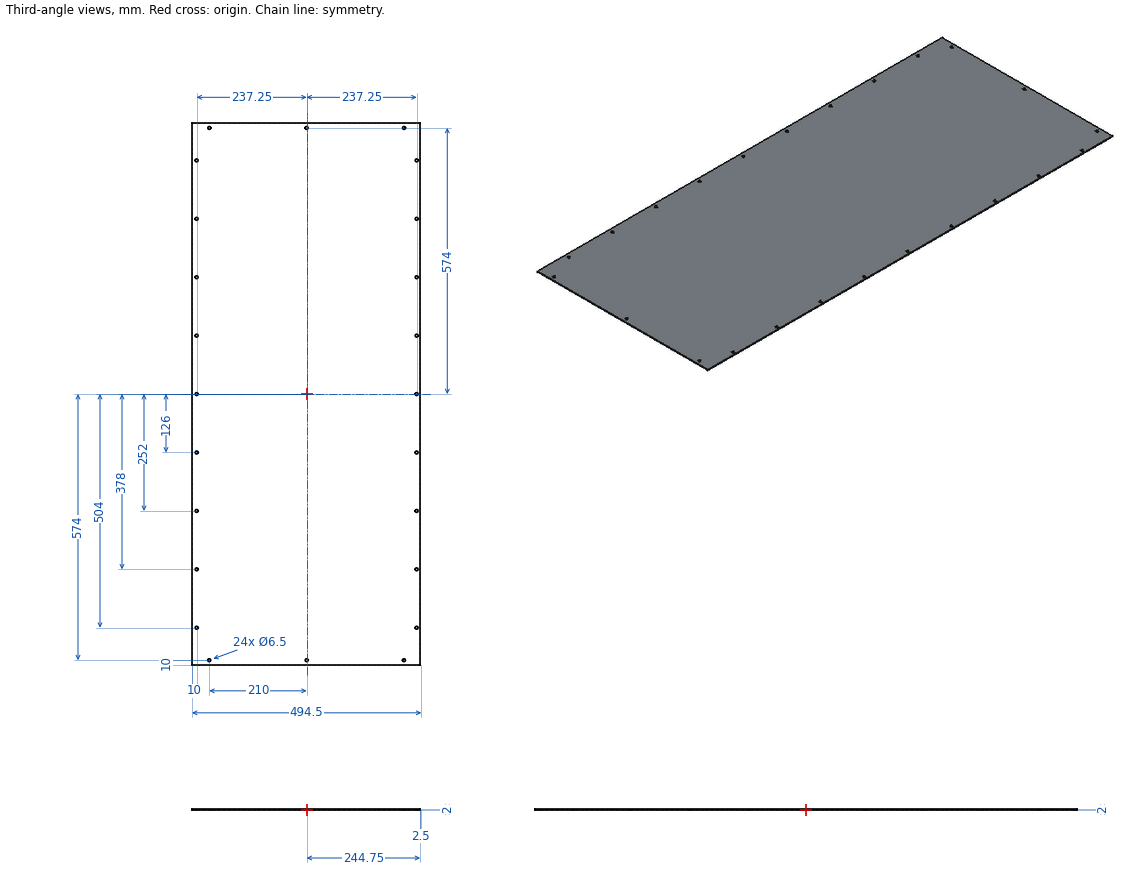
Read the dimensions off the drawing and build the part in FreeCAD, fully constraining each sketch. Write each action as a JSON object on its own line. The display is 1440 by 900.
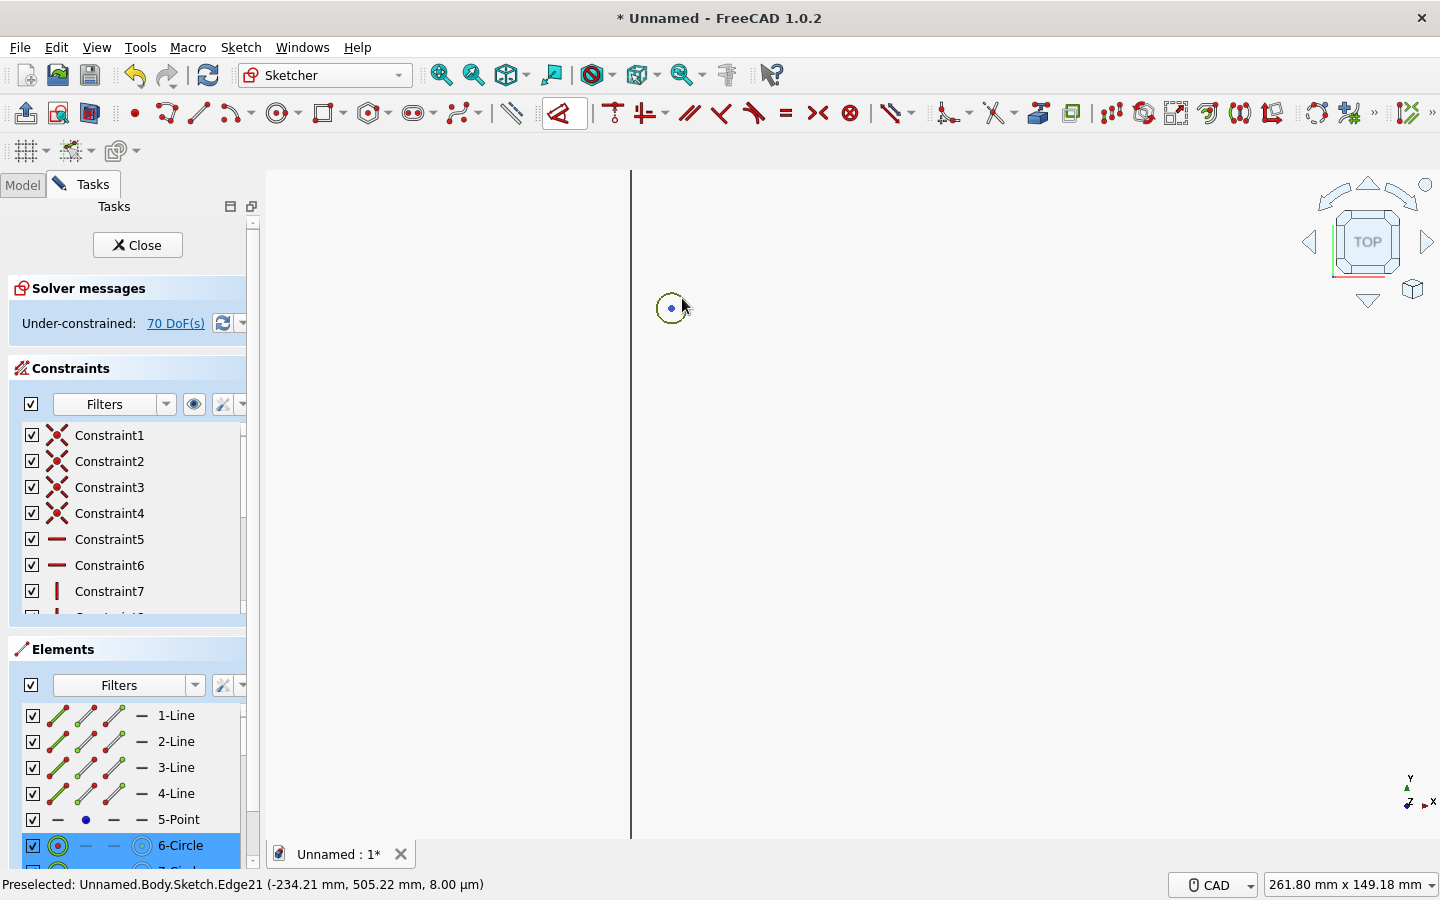
{"action": "scroll", "coordinate": [690, 299], "scroll_direction": "down", "scroll_amount": 12}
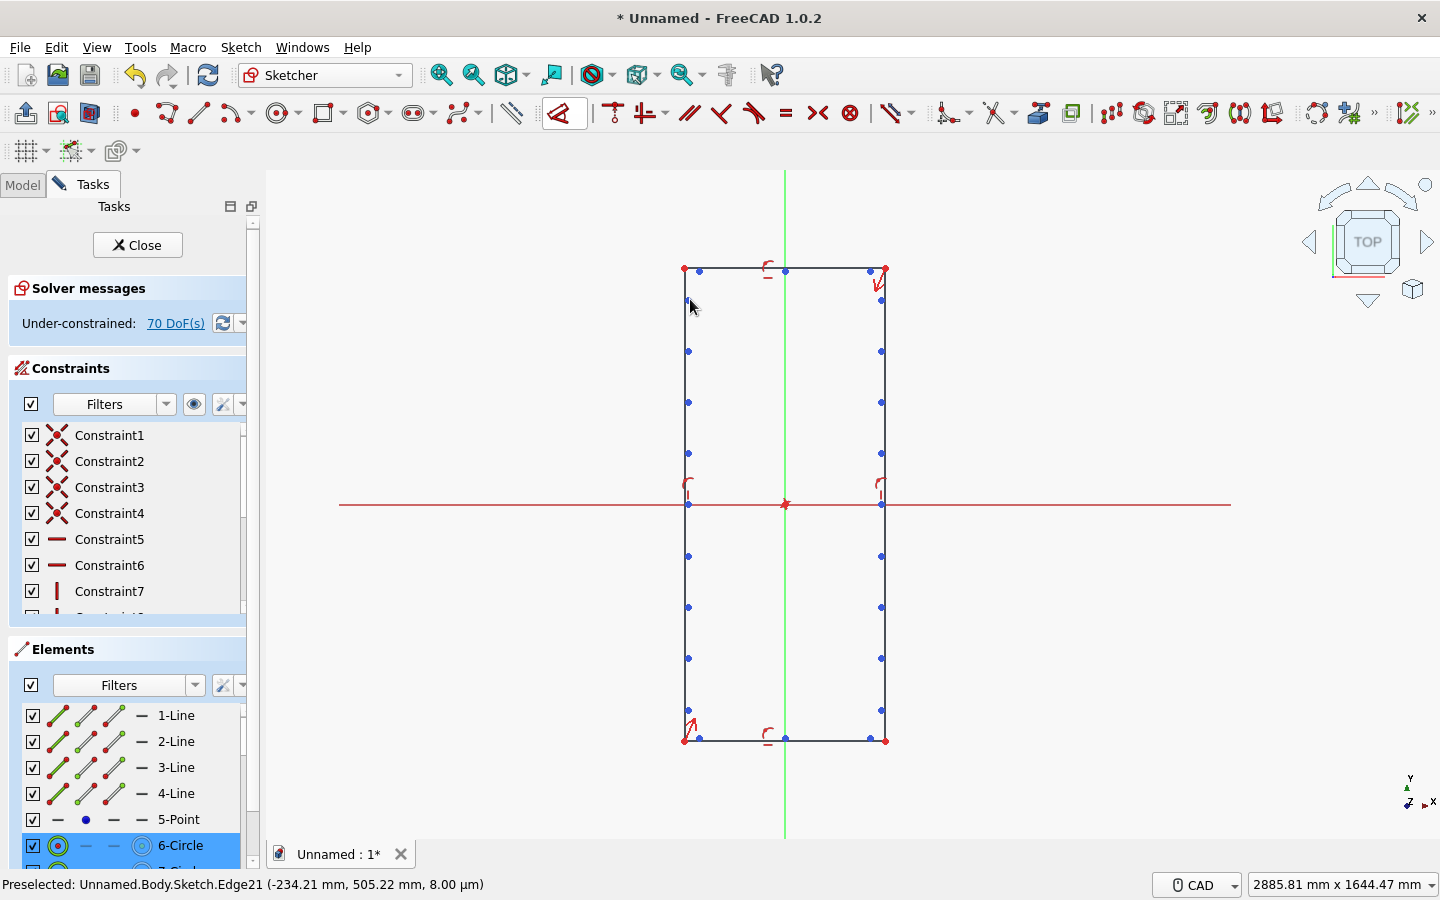
{"action": "scroll", "coordinate": [701, 271], "scroll_direction": "up", "scroll_amount": 12}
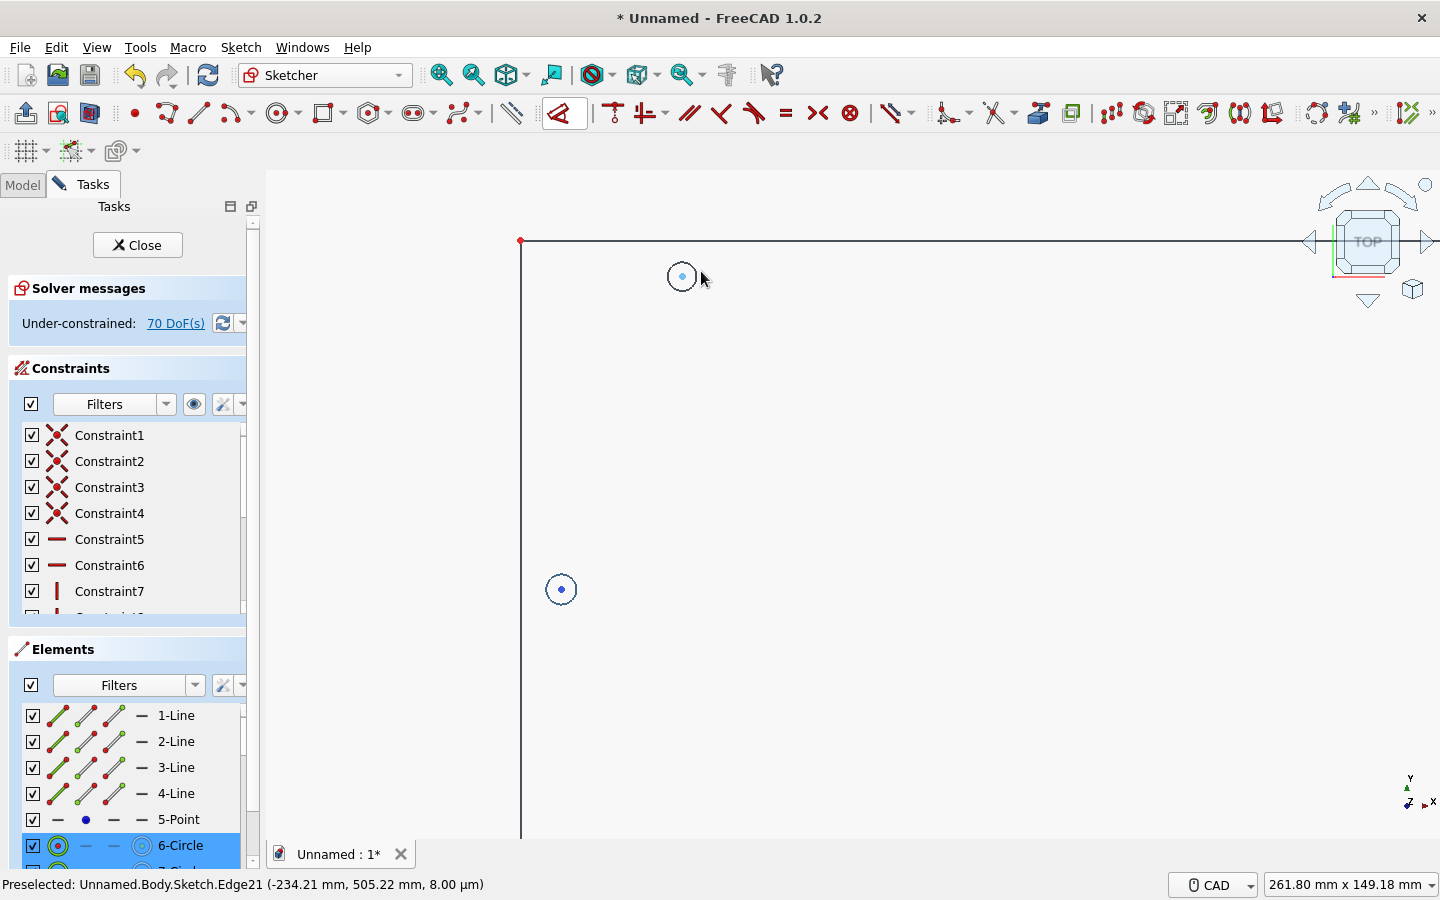
{"action": "left_click", "coordinate": [692, 266]}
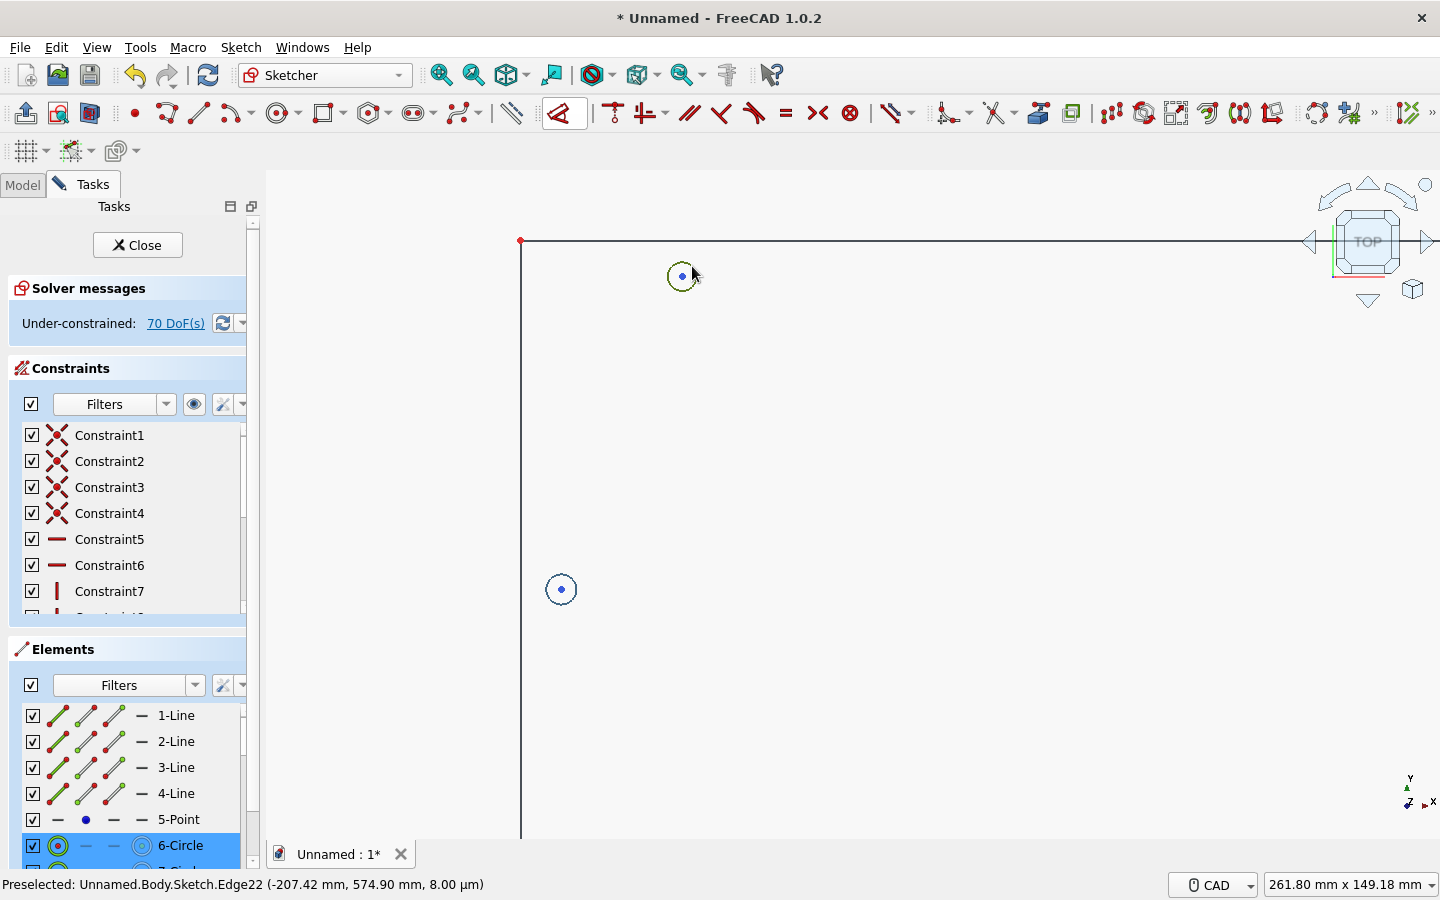
{"action": "scroll", "coordinate": [701, 271], "scroll_direction": "down", "scroll_amount": 12}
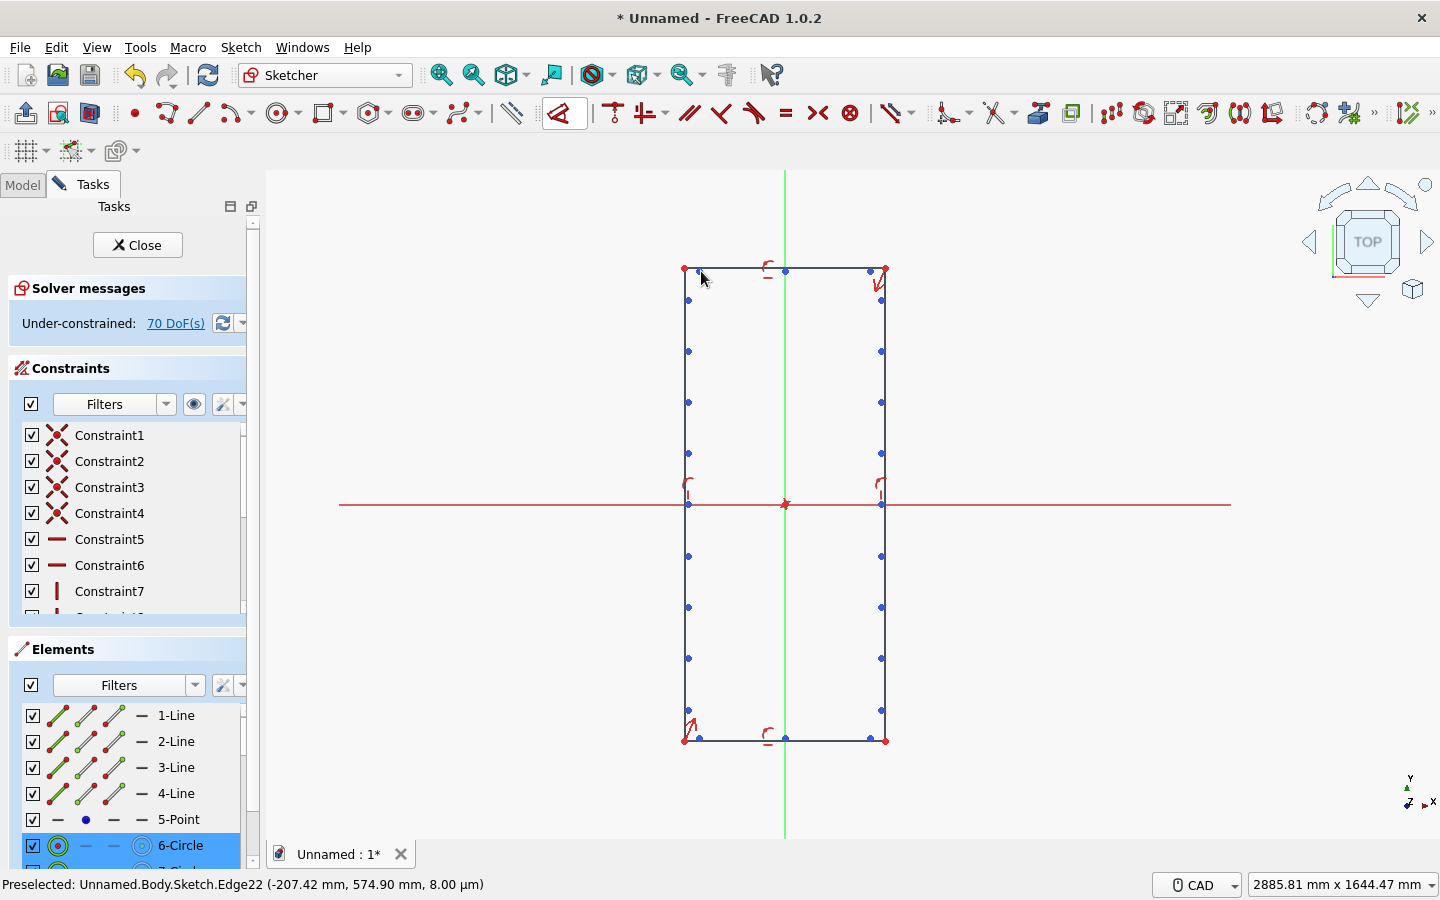
{"action": "scroll", "coordinate": [883, 504], "scroll_direction": "up", "scroll_amount": 14}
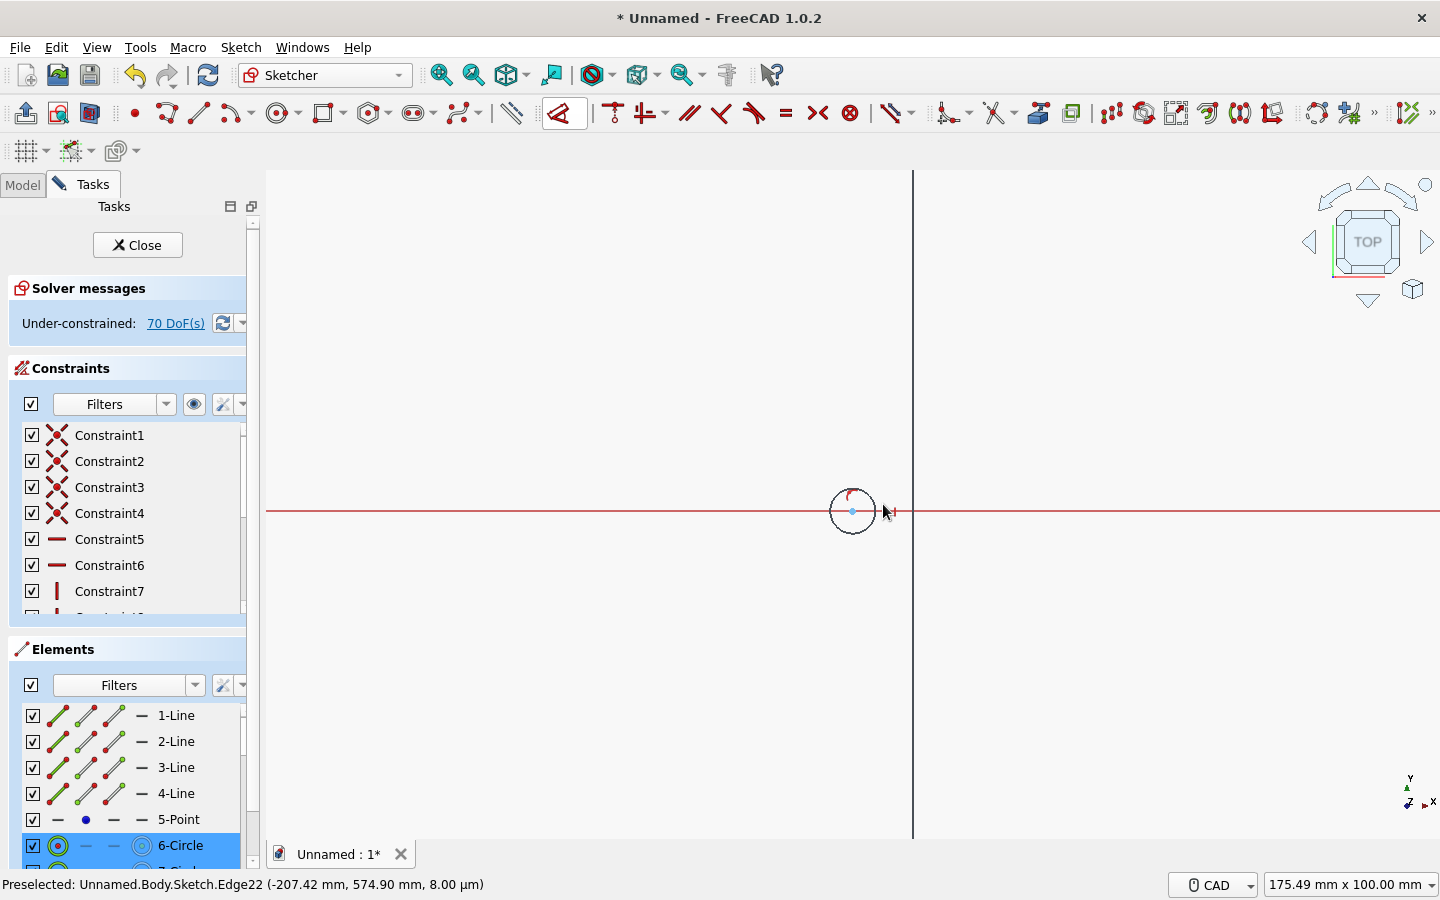
{"action": "left_click", "coordinate": [869, 495]}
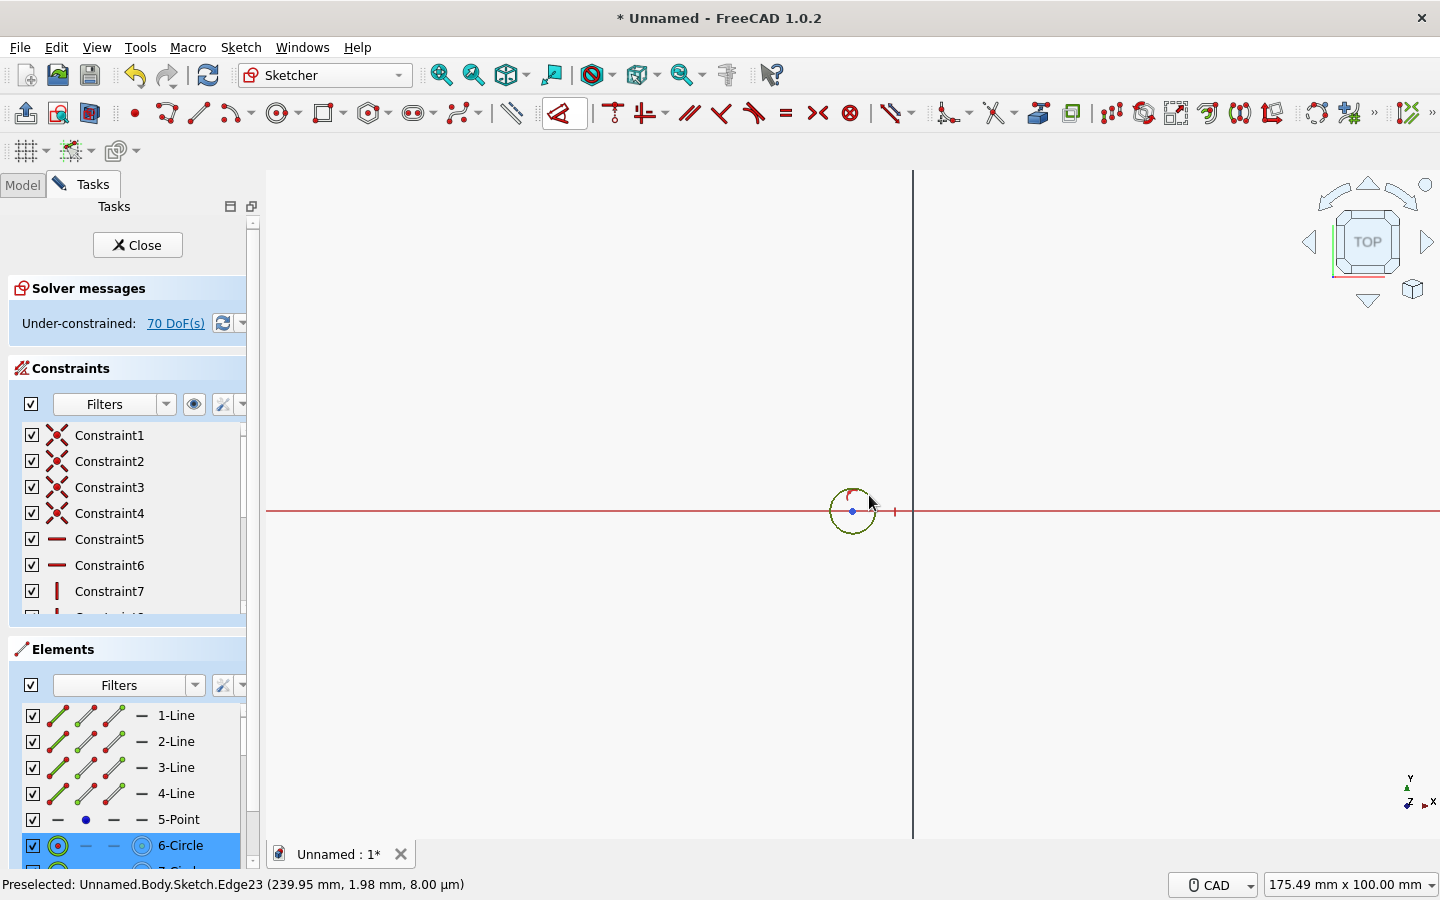
{"action": "scroll", "coordinate": [883, 504], "scroll_direction": "down", "scroll_amount": 14}